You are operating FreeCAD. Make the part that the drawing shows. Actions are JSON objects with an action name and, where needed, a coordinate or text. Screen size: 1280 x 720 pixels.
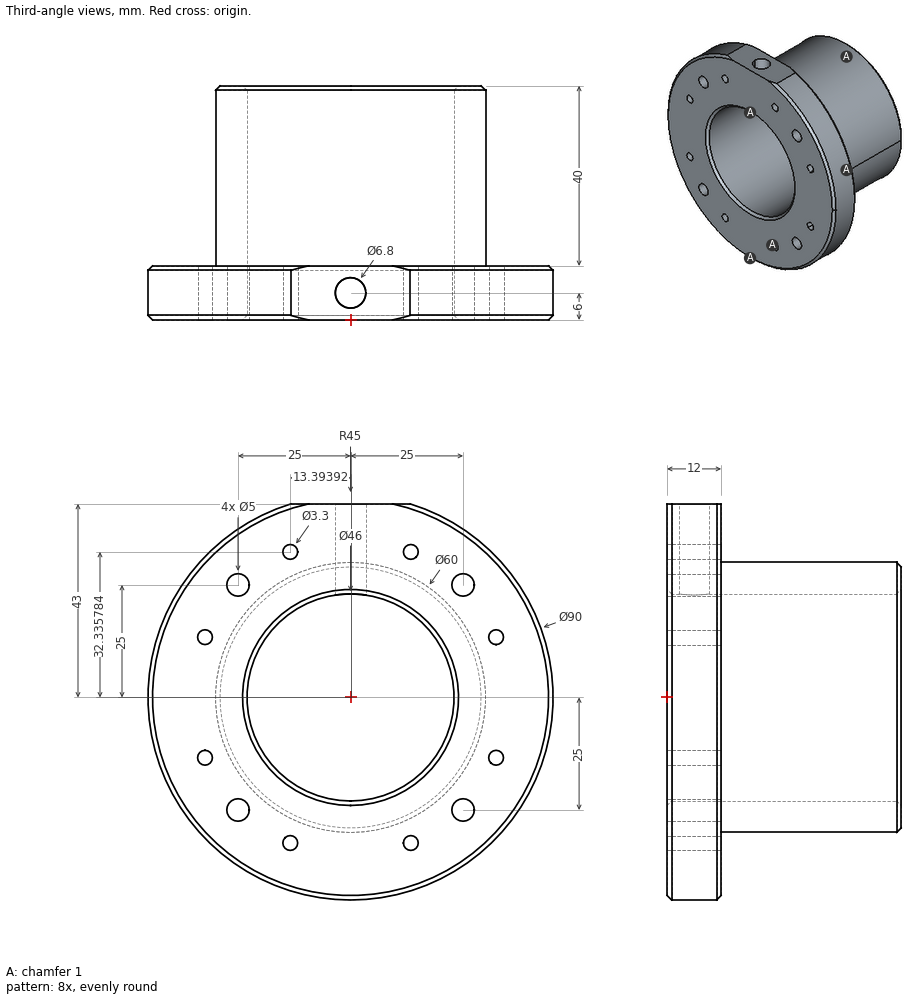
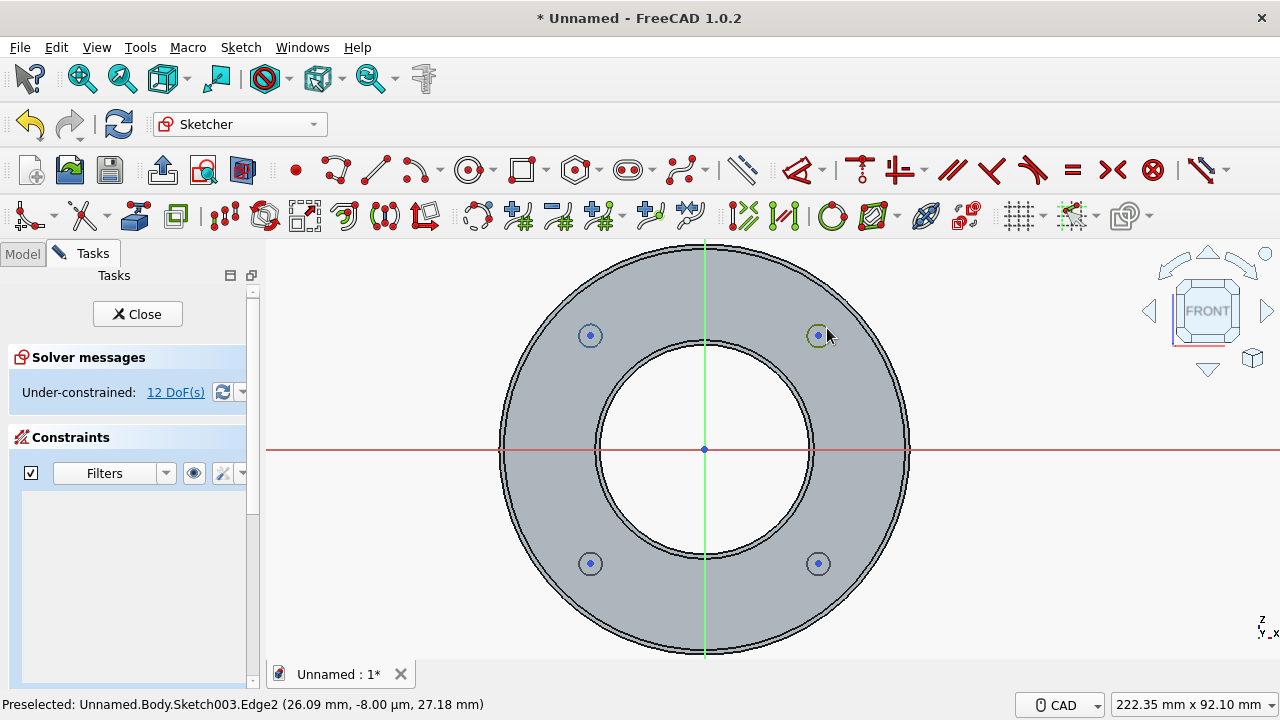
{"action": "left_click", "coordinate": [826, 556]}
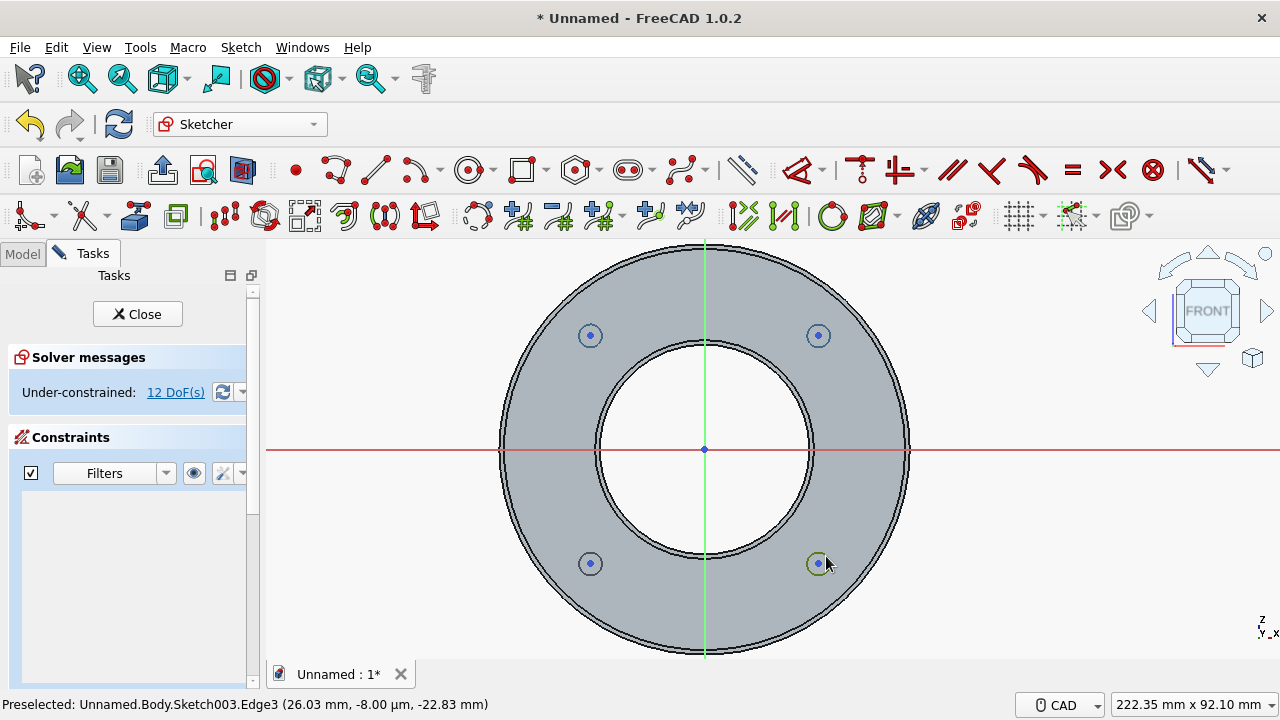
{"action": "left_click", "coordinate": [599, 556]}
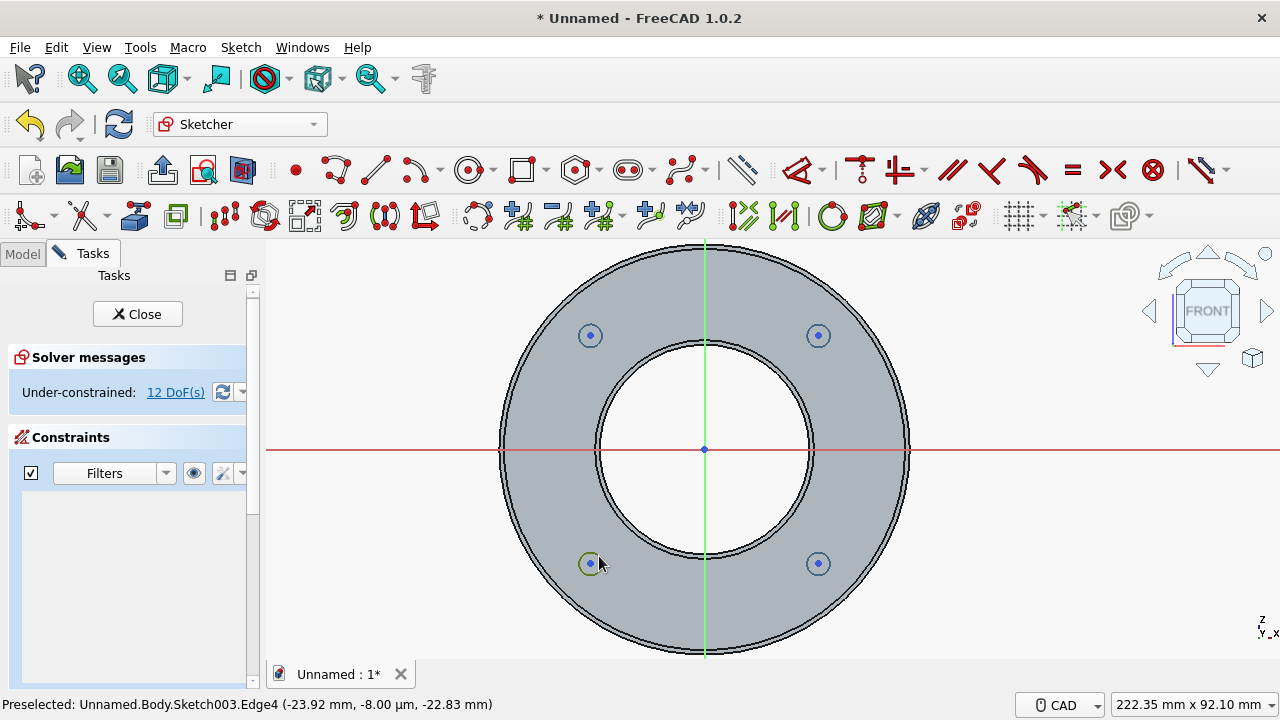
{"action": "key", "text": "e"}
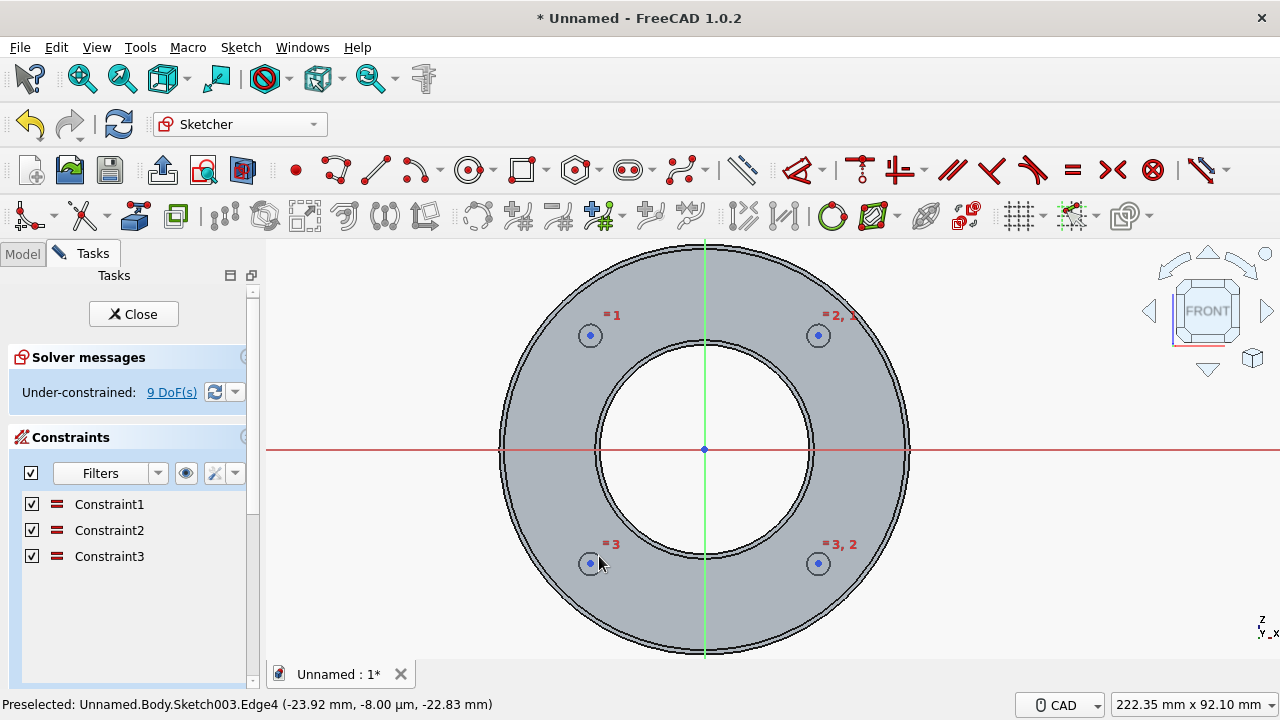
{"action": "left_click", "coordinate": [590, 336]}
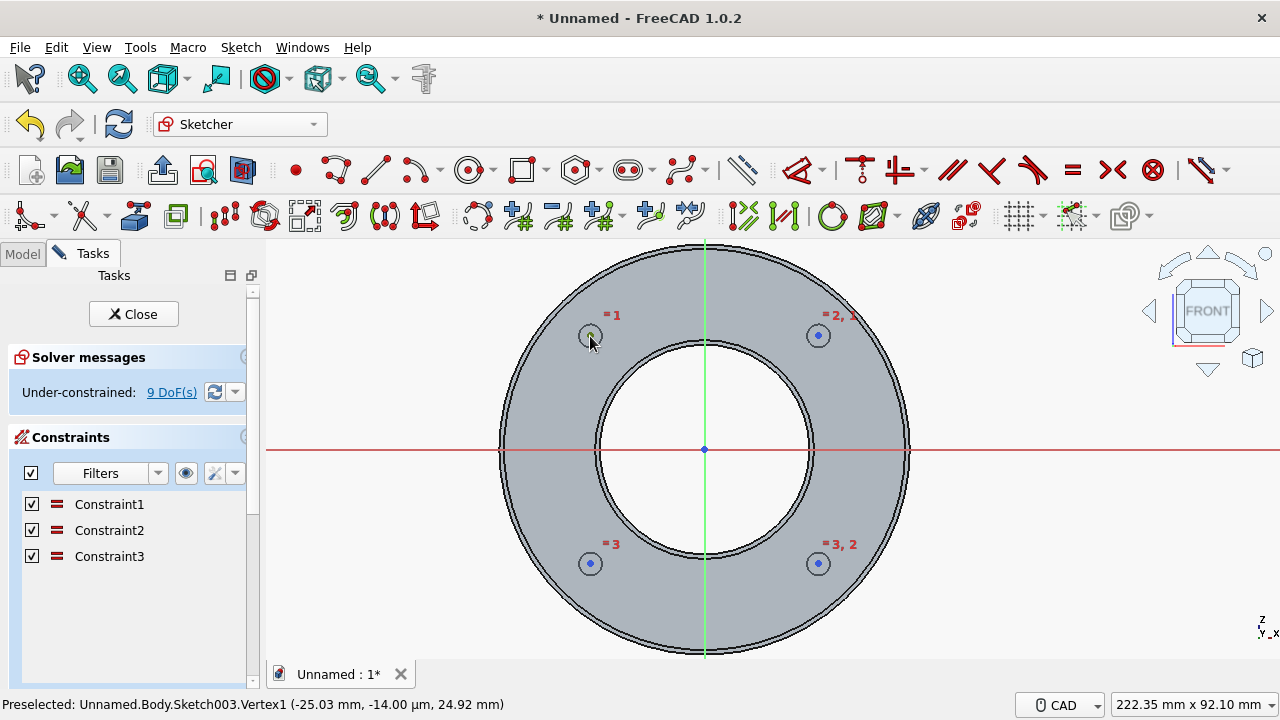
{"action": "left_click", "coordinate": [819, 336]}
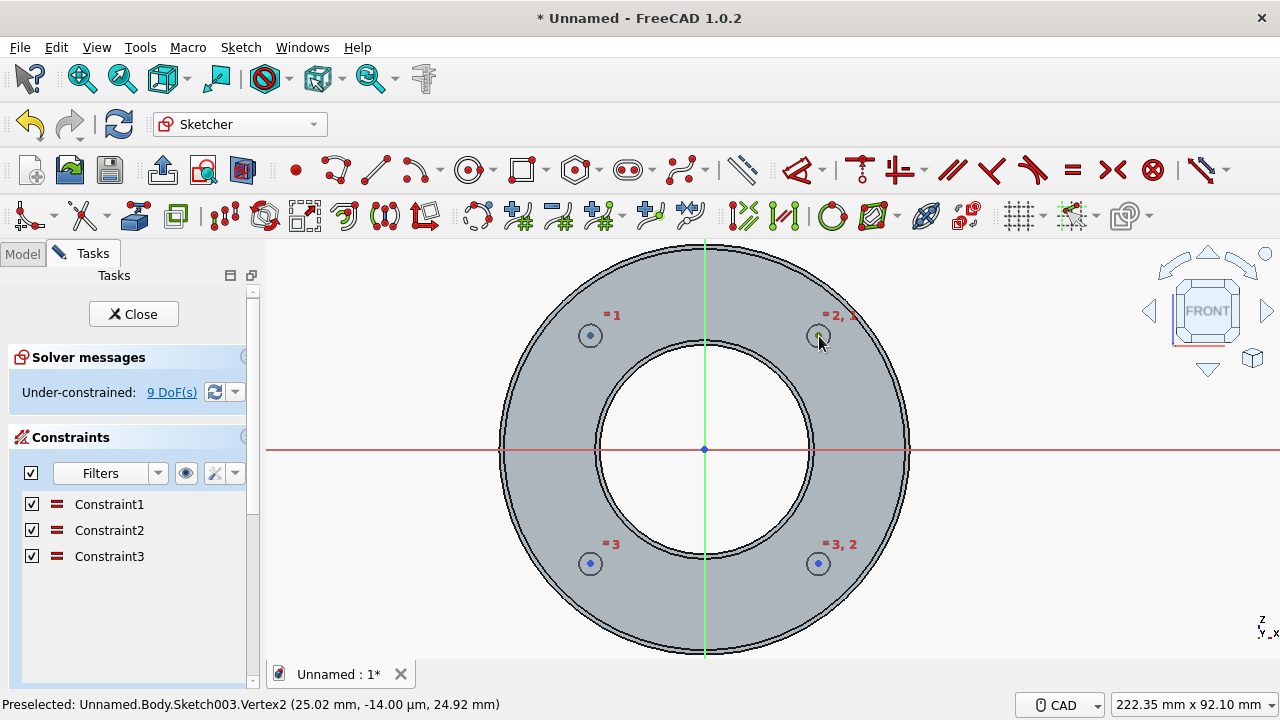
{"action": "key", "text": "h"}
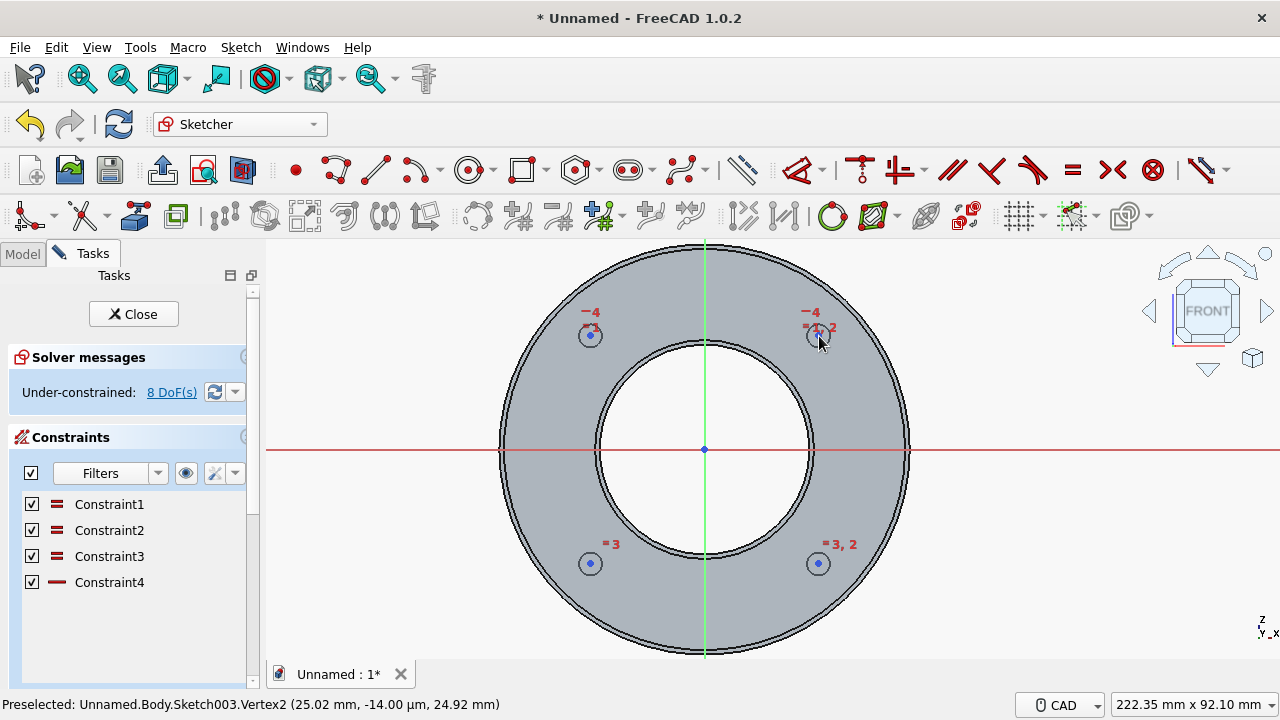
{"action": "left_click", "coordinate": [819, 336]}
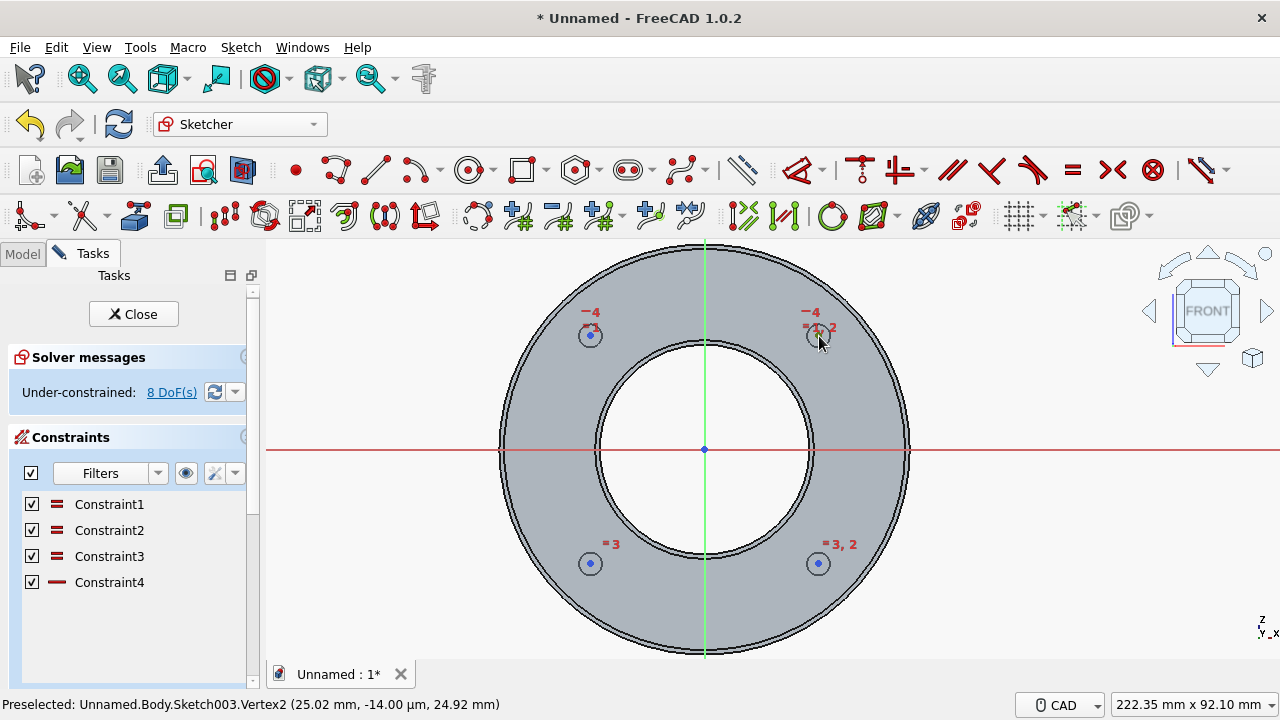
{"action": "left_click", "coordinate": [818, 564]}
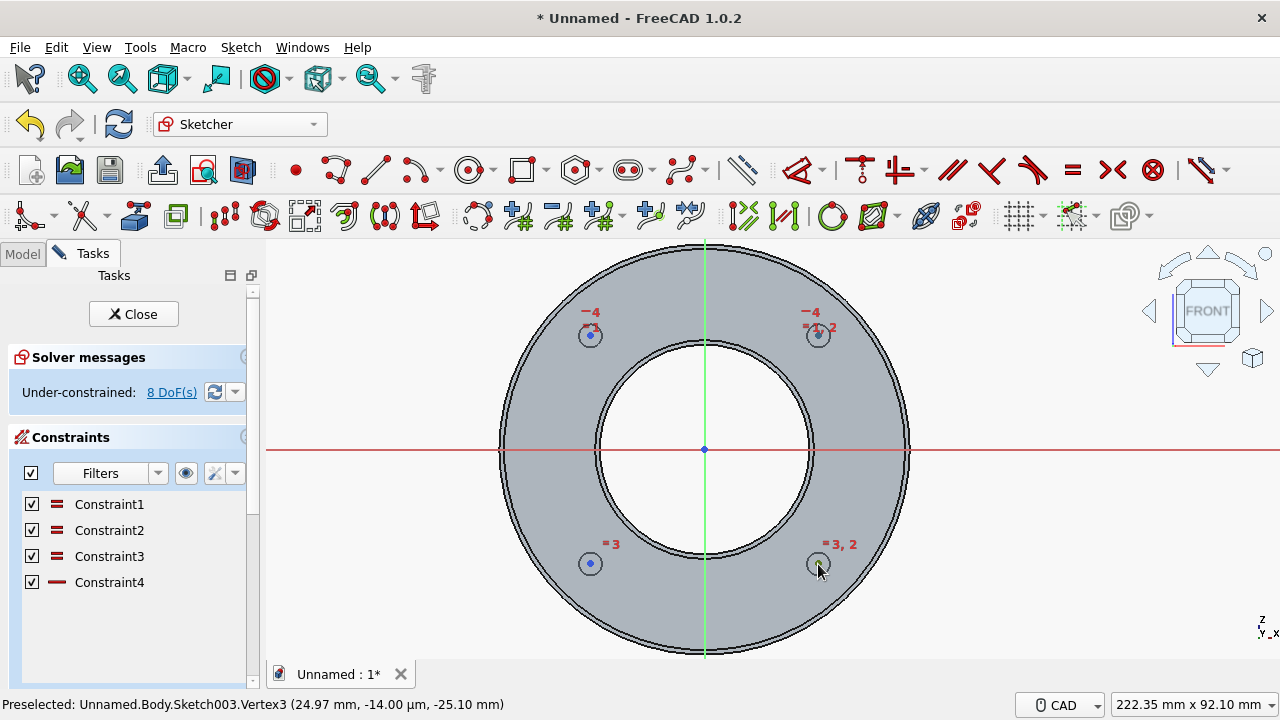
{"action": "key", "text": "v"}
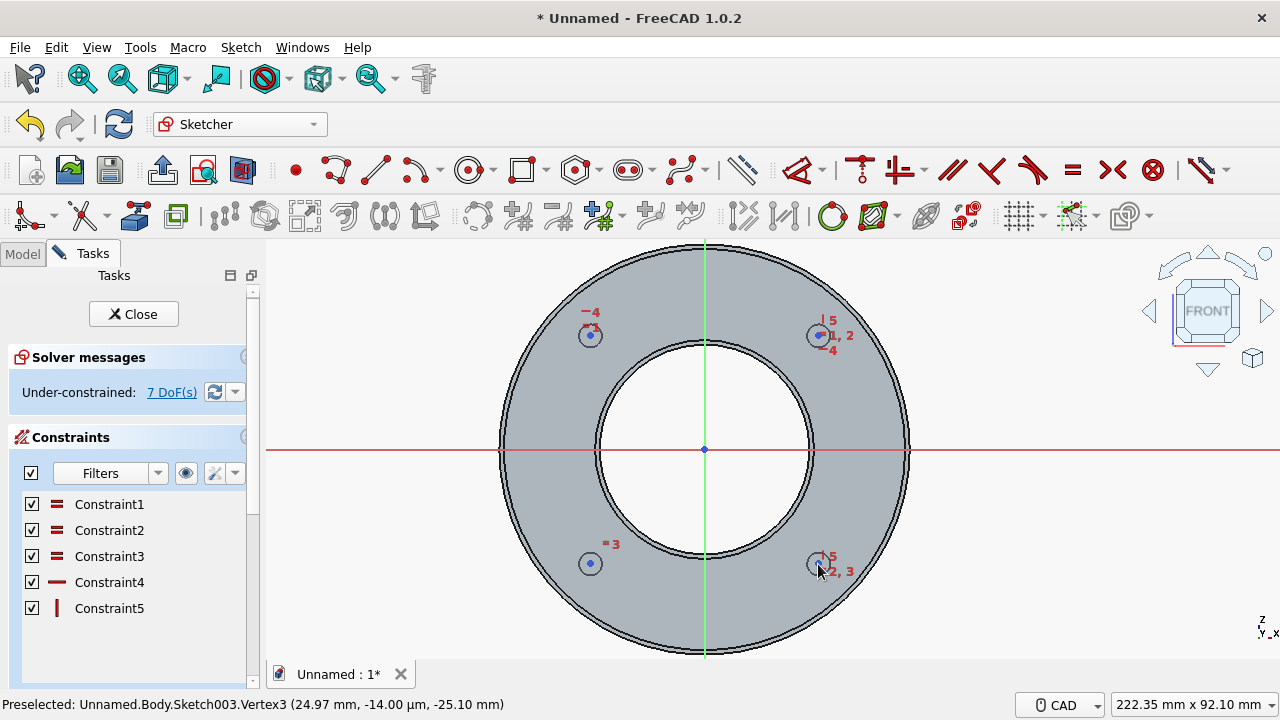
{"action": "left_click", "coordinate": [590, 336]}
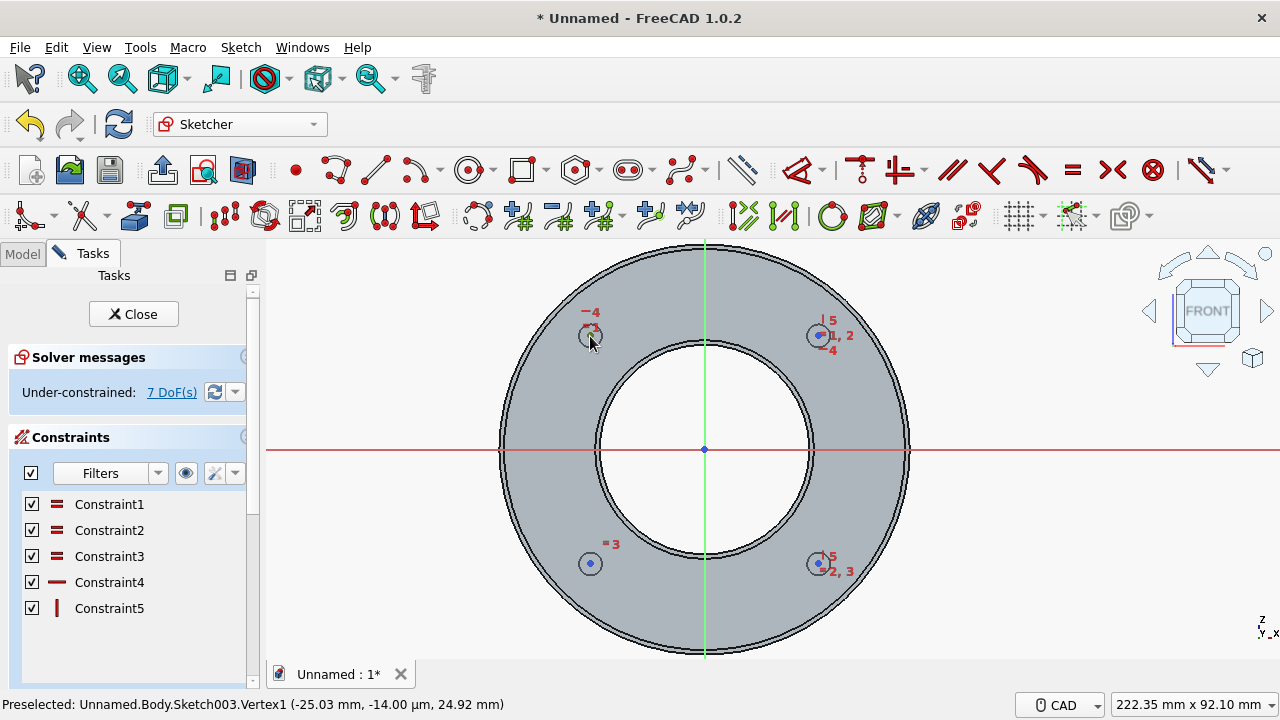
{"action": "left_click", "coordinate": [591, 564]}